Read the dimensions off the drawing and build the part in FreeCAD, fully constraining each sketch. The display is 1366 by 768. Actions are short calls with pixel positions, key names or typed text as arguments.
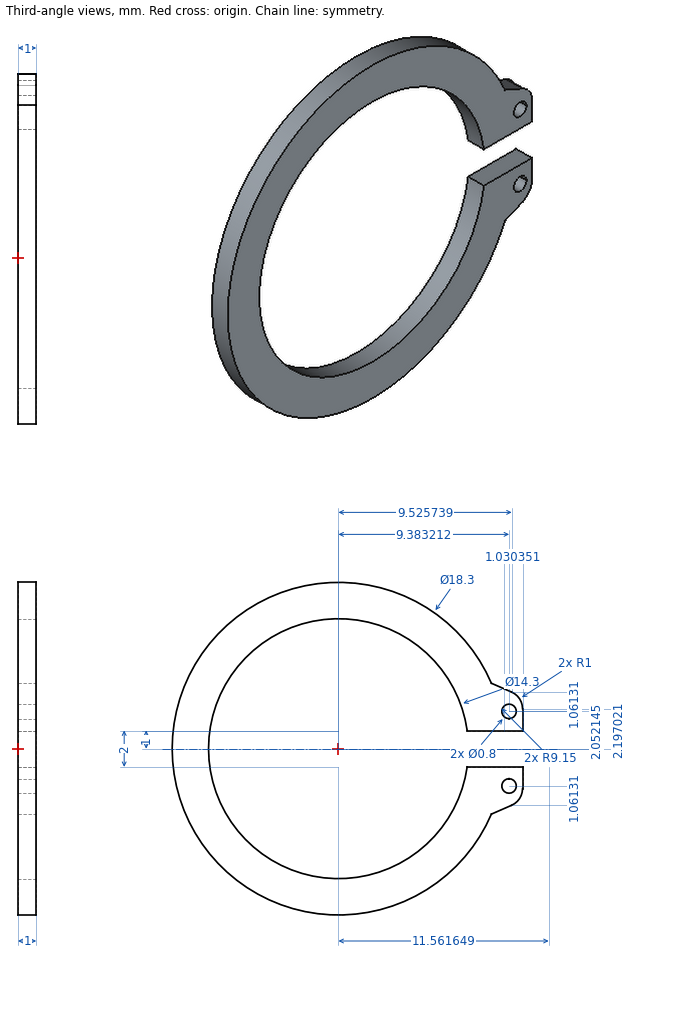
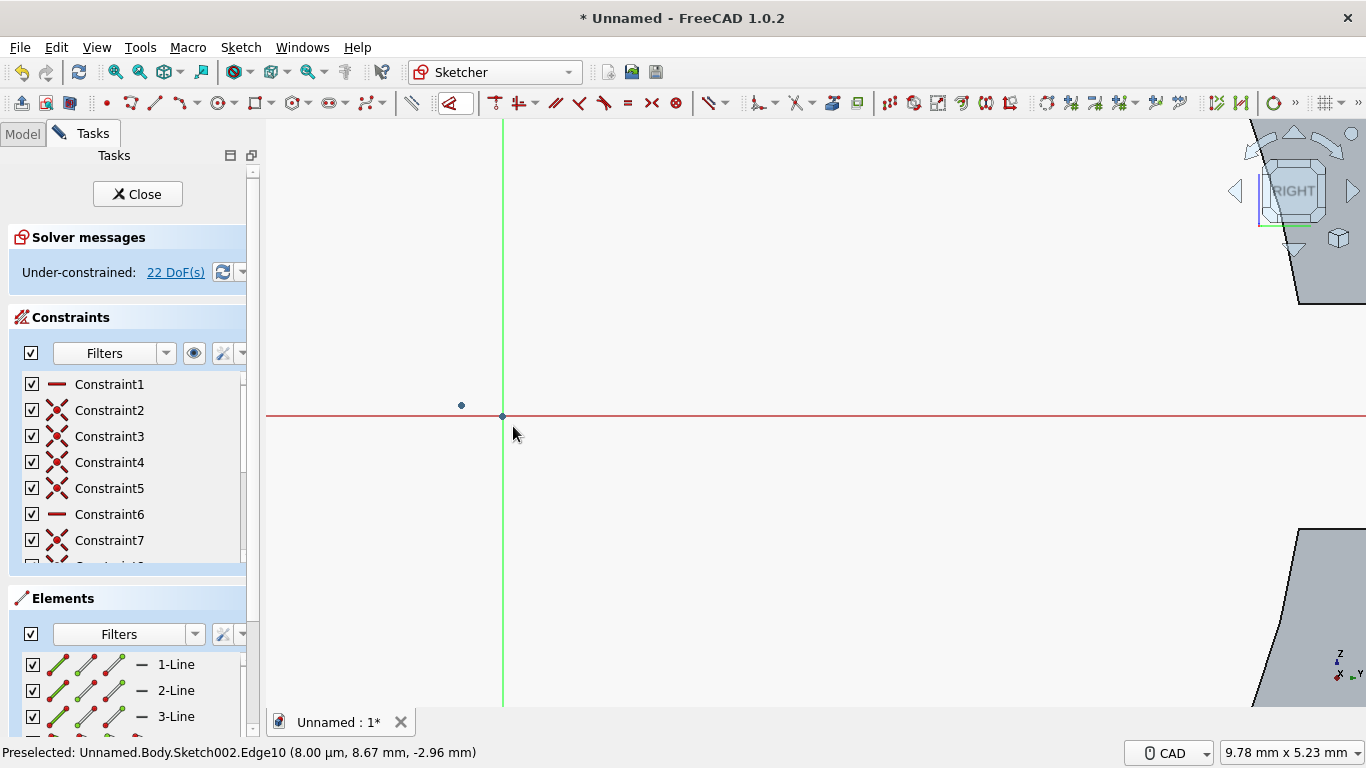
key(c)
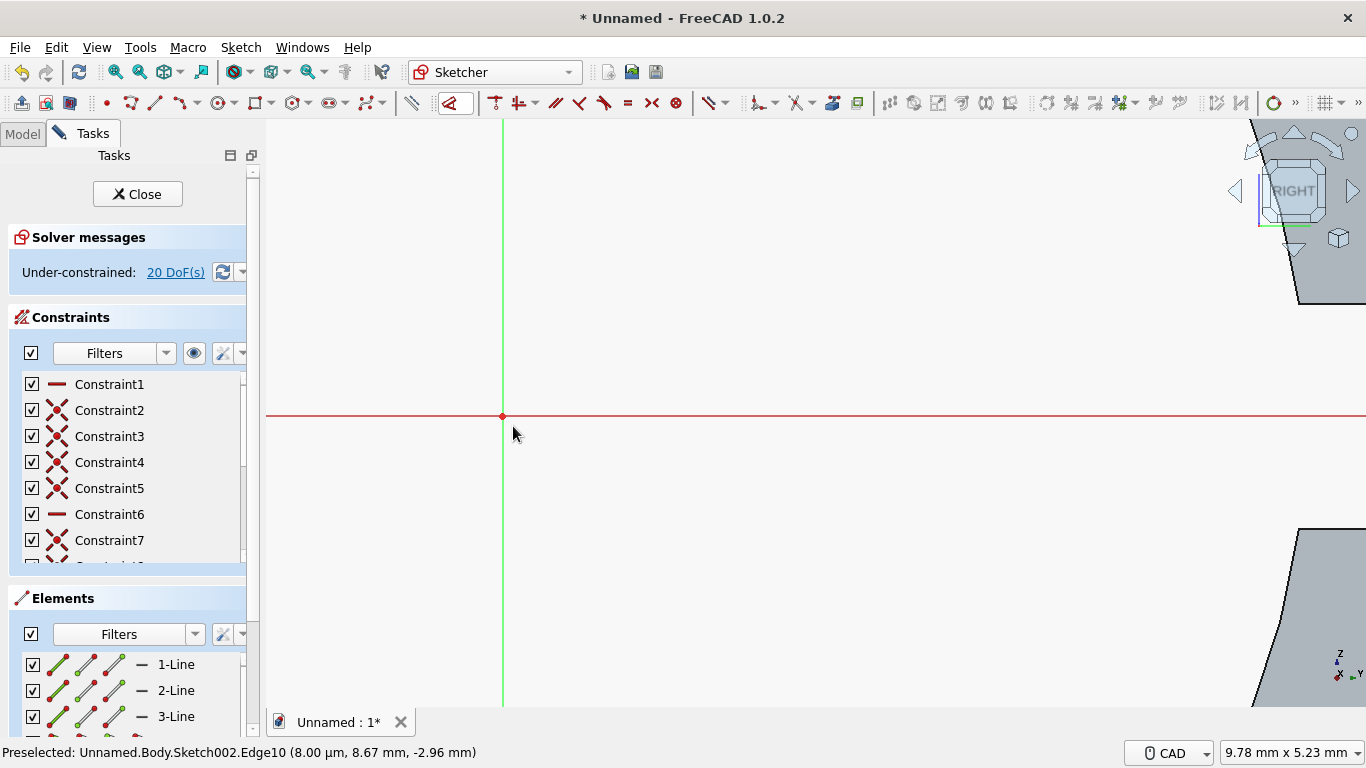
scroll(483, 411, down, 4)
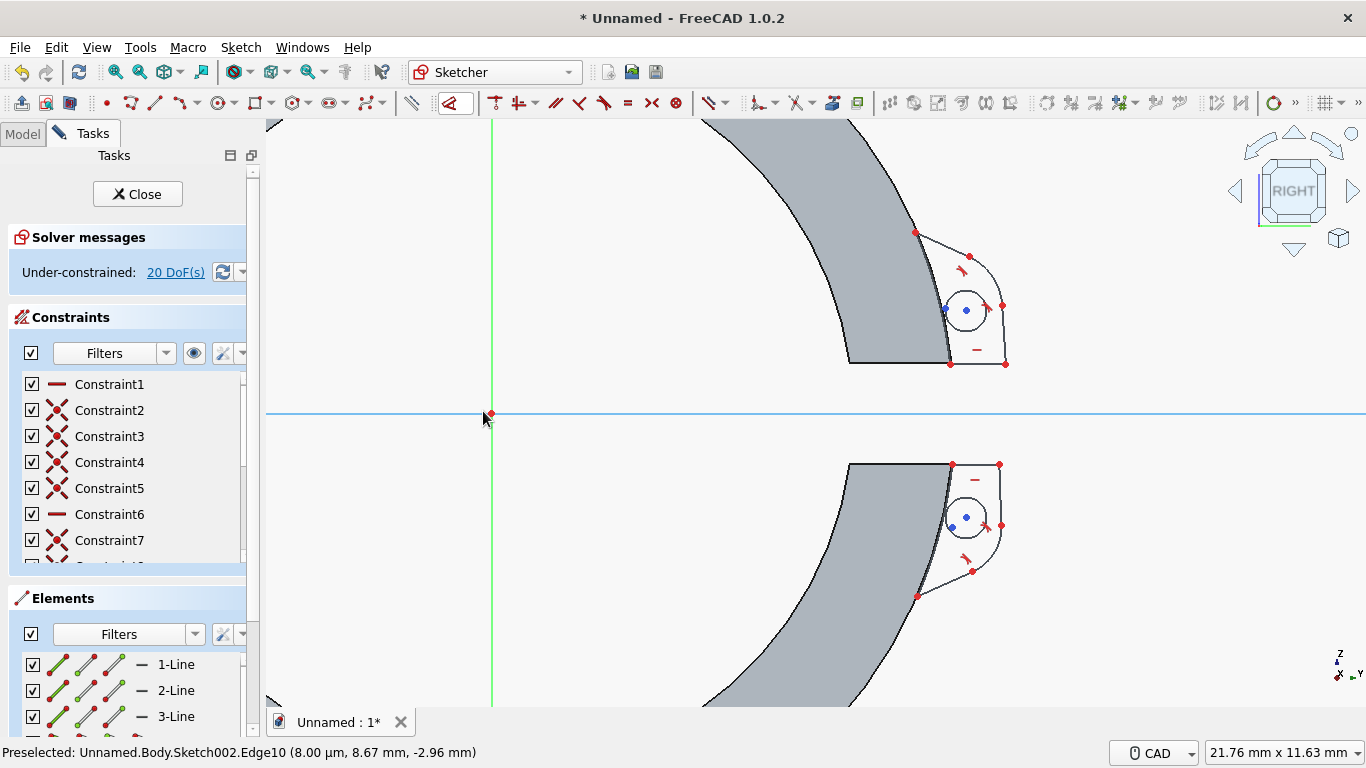
click(998, 287)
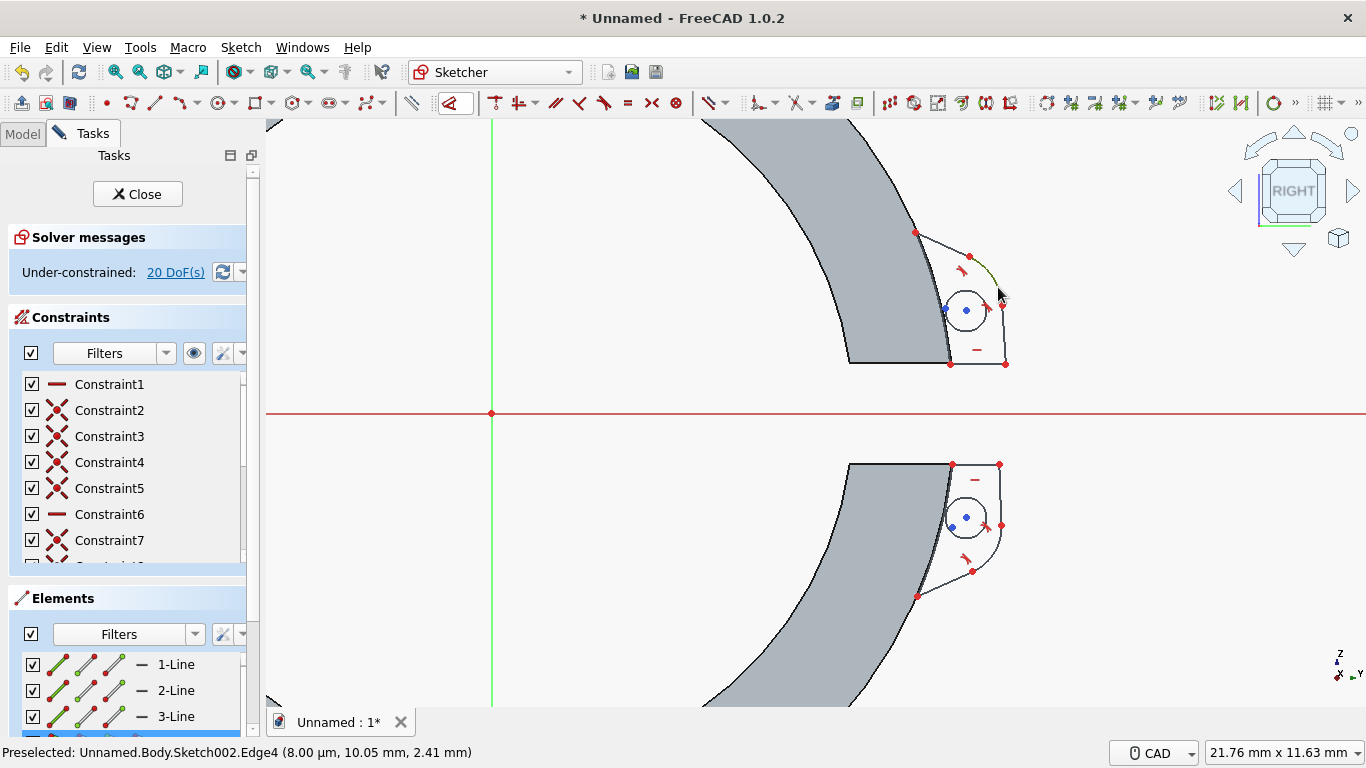
click(987, 562)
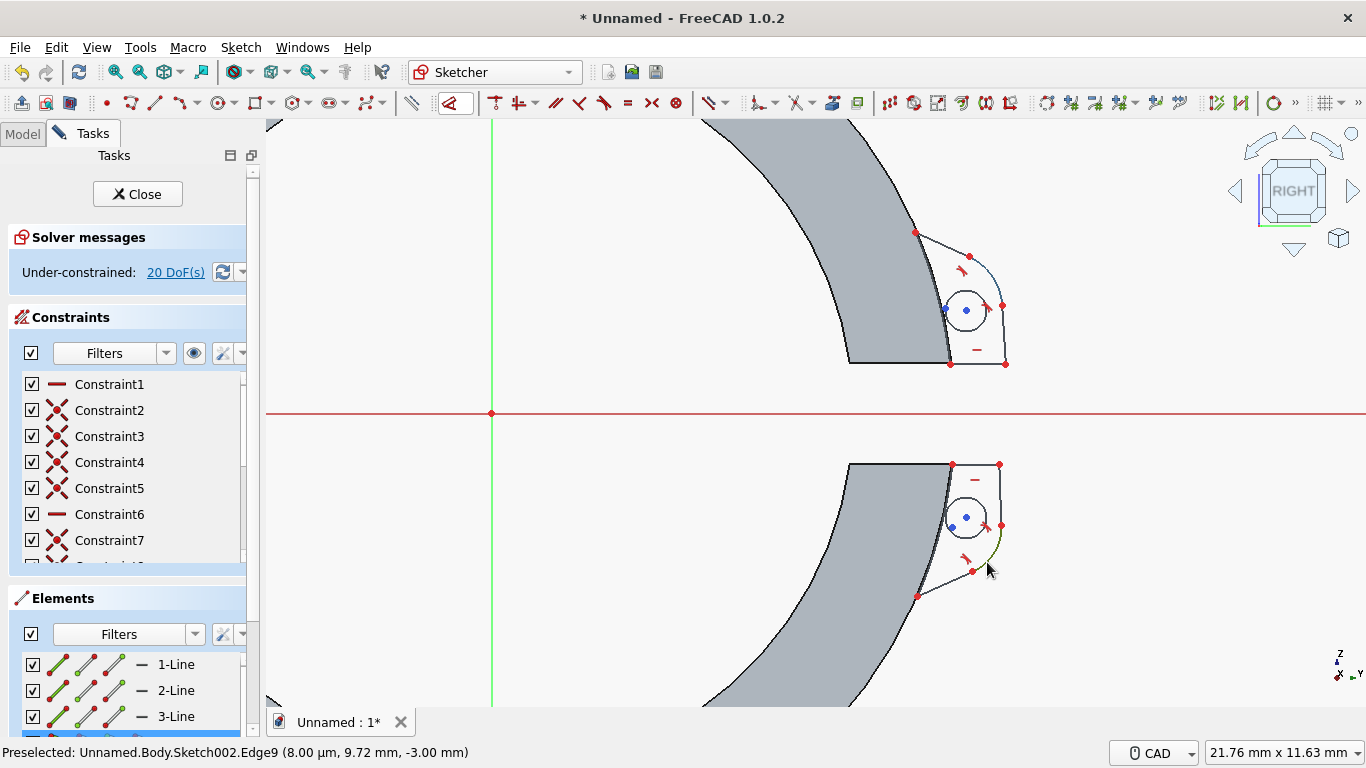
click(628, 104)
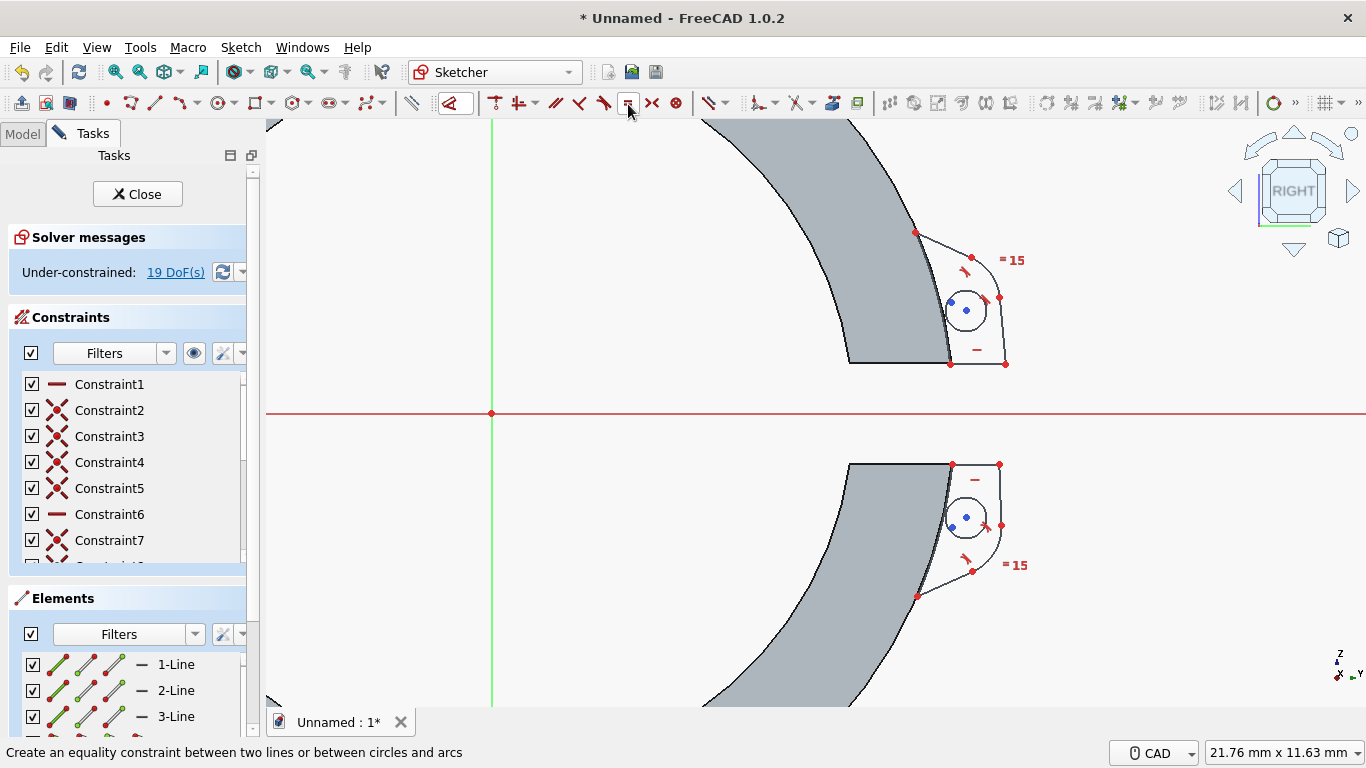
click(930, 271)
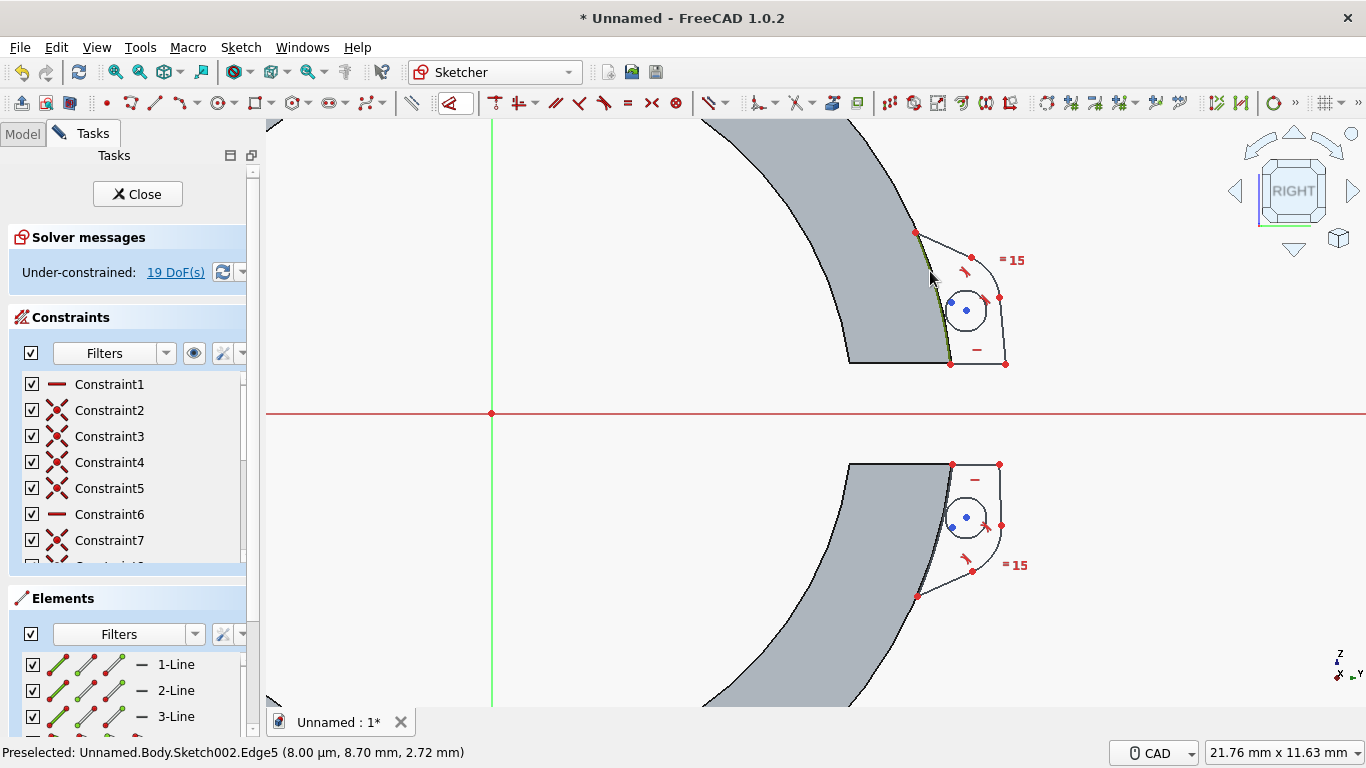
click(932, 558)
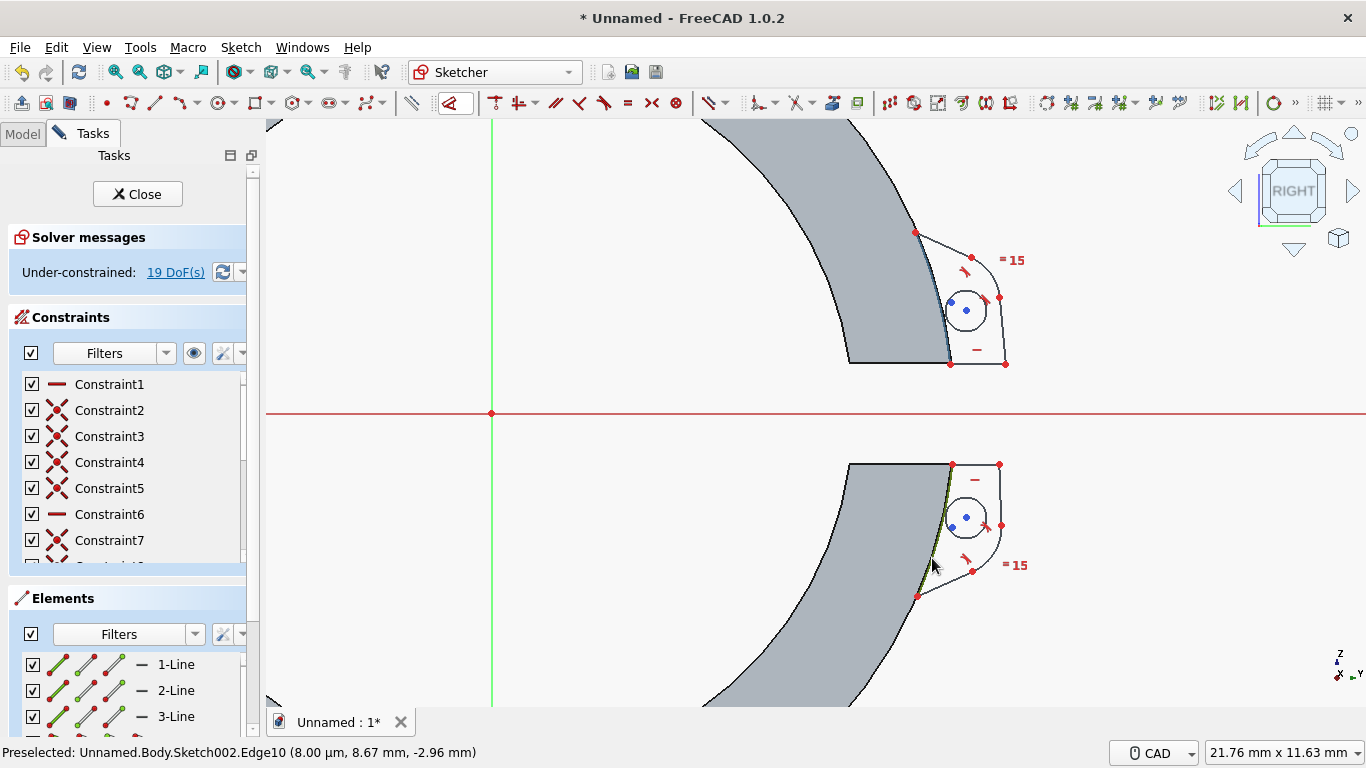
click(628, 104)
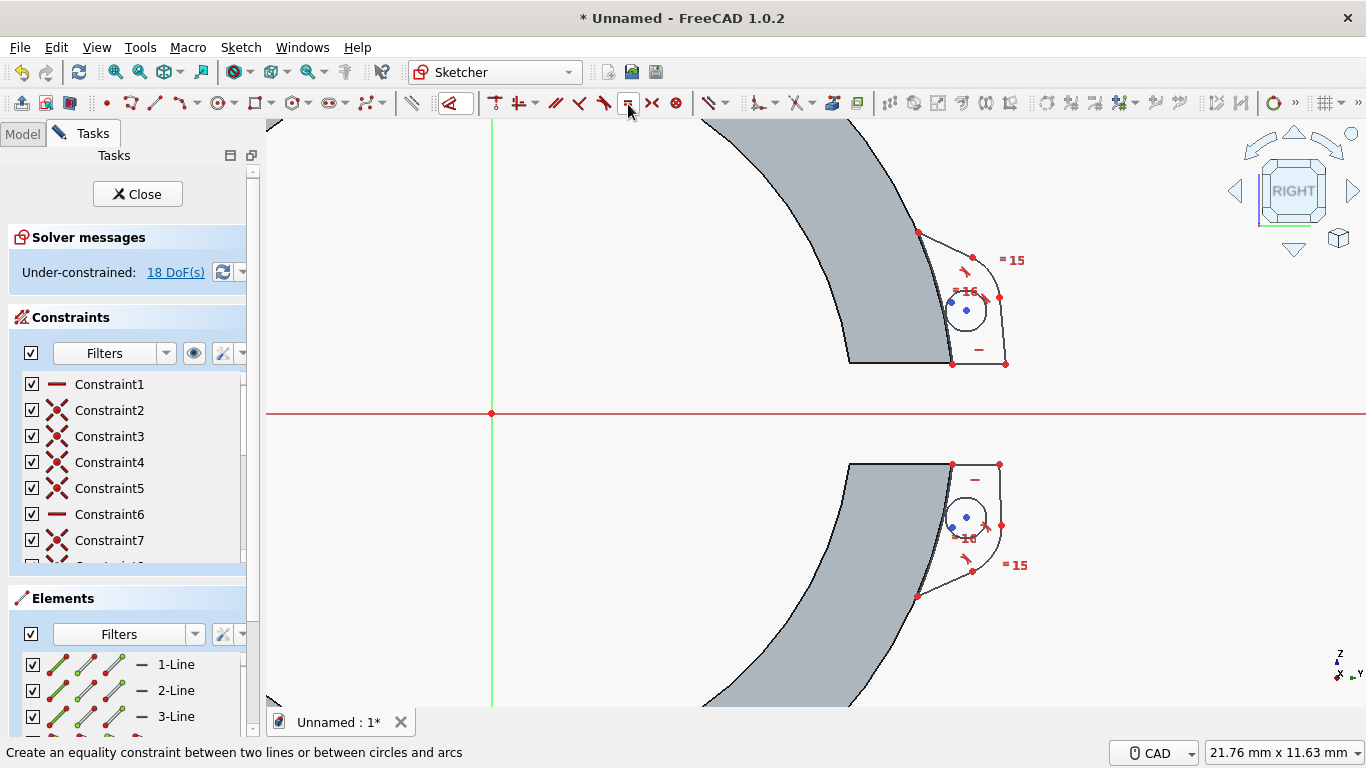
click(981, 325)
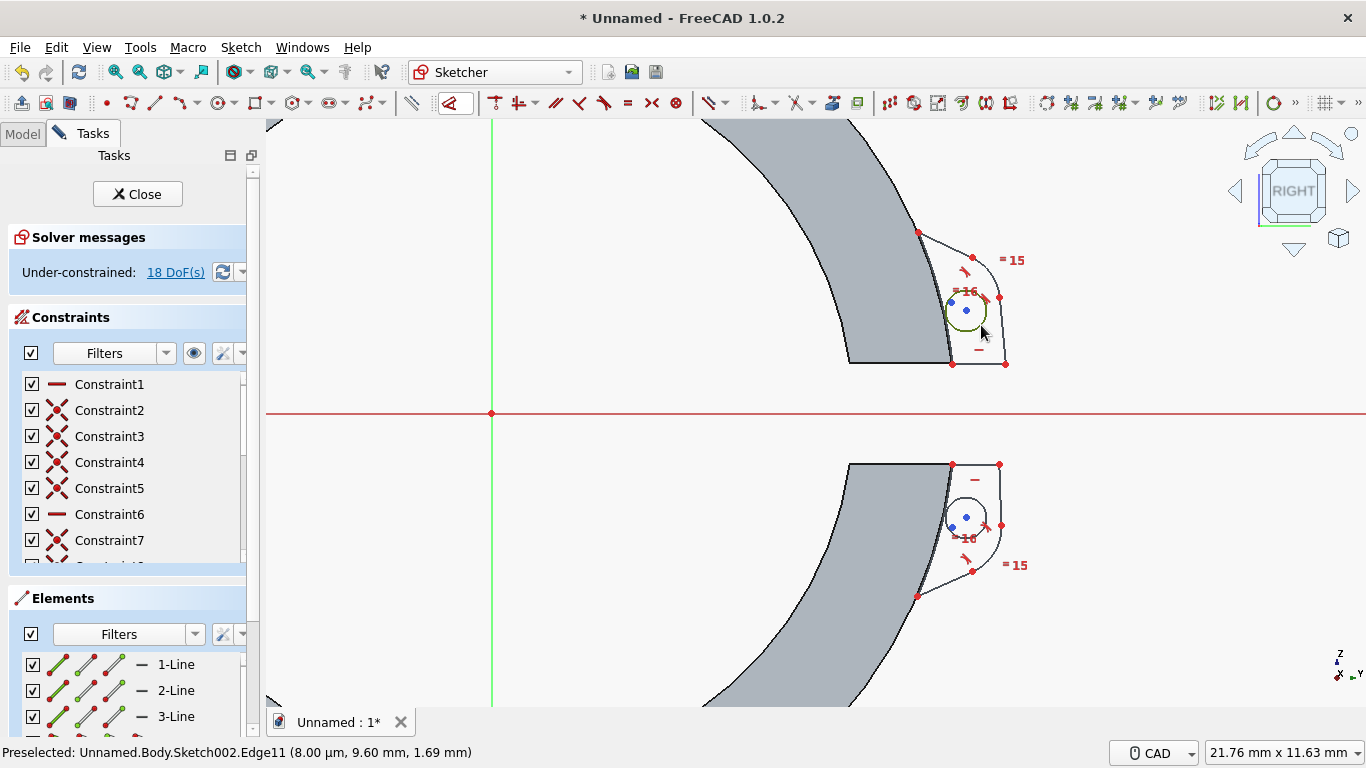
click(980, 503)